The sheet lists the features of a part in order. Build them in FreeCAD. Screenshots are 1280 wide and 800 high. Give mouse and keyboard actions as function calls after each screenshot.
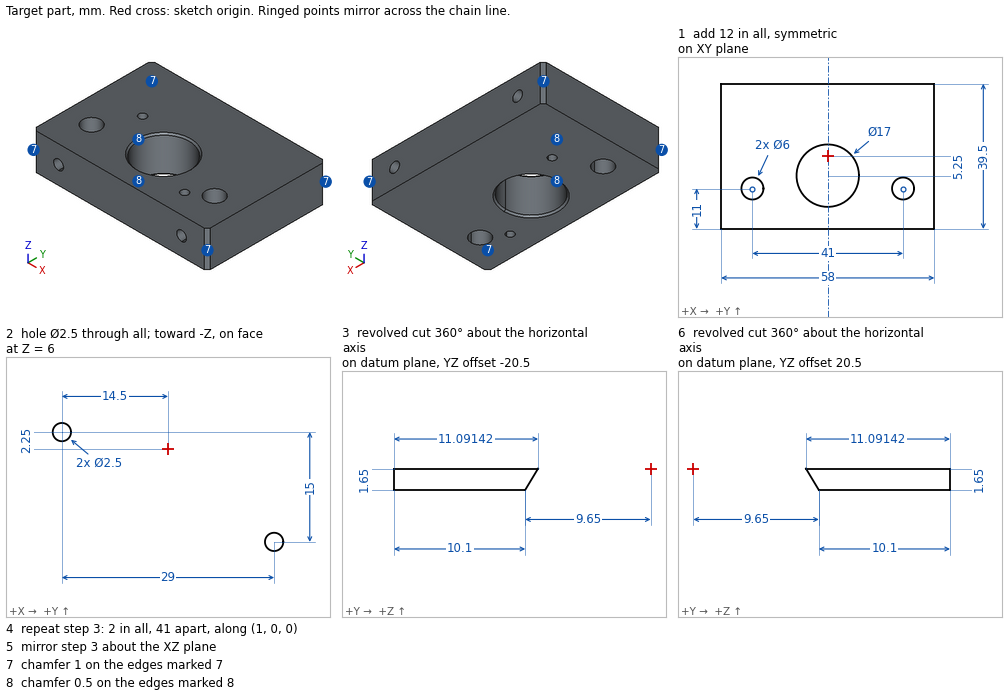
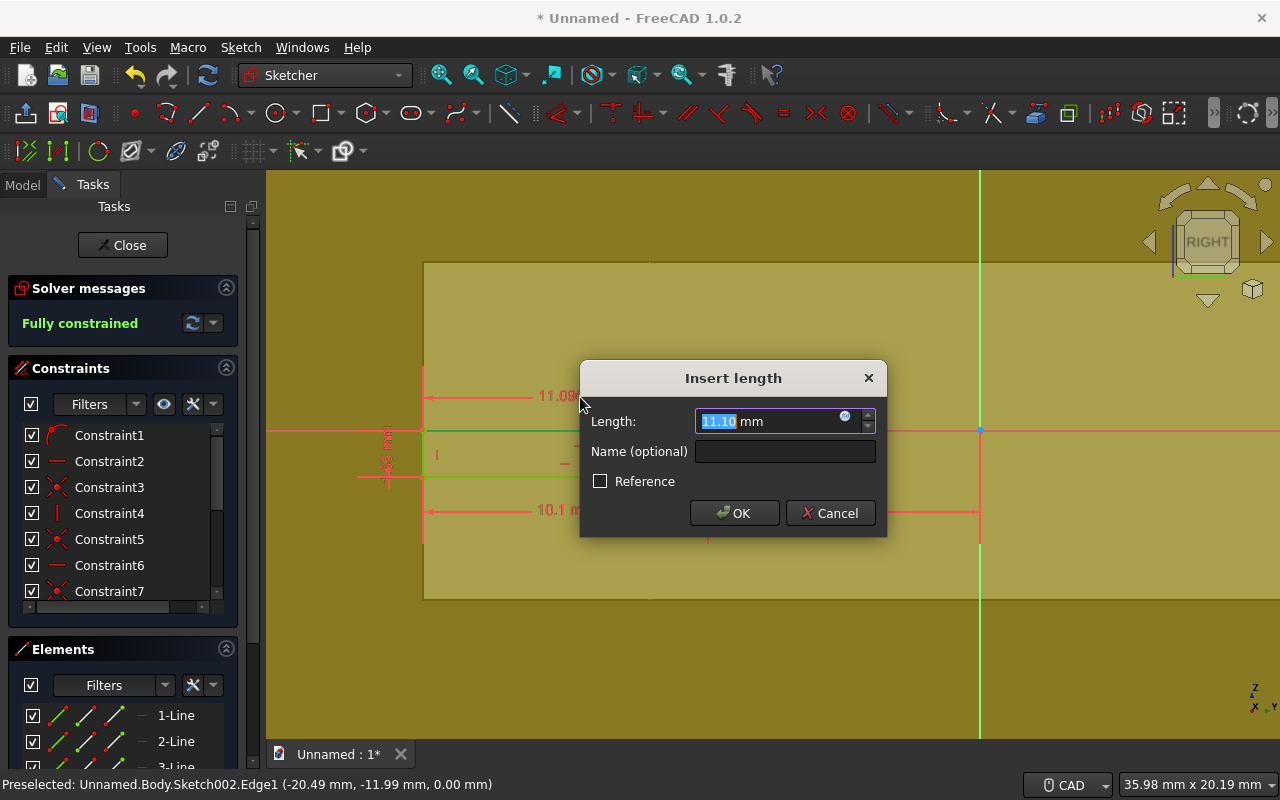
text(11.09142)
key(Return)
key(Escape)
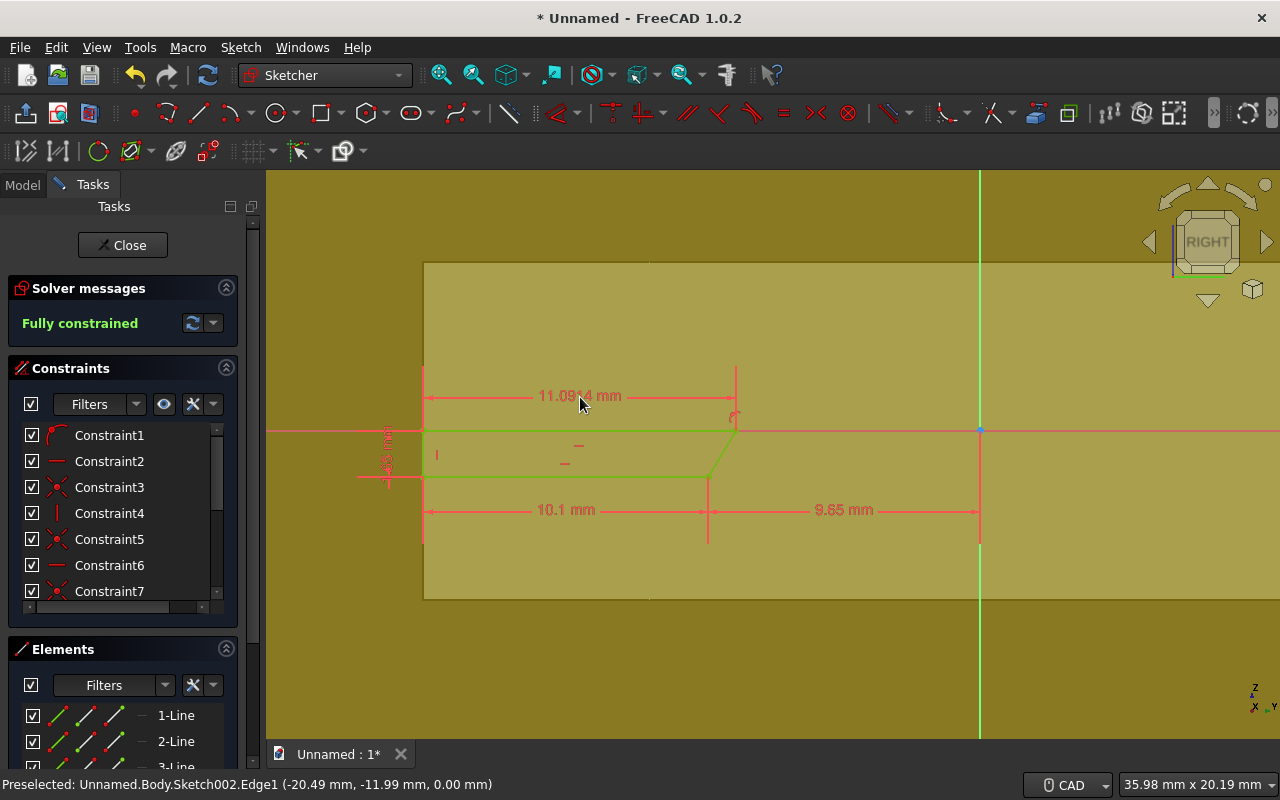
click(123, 245)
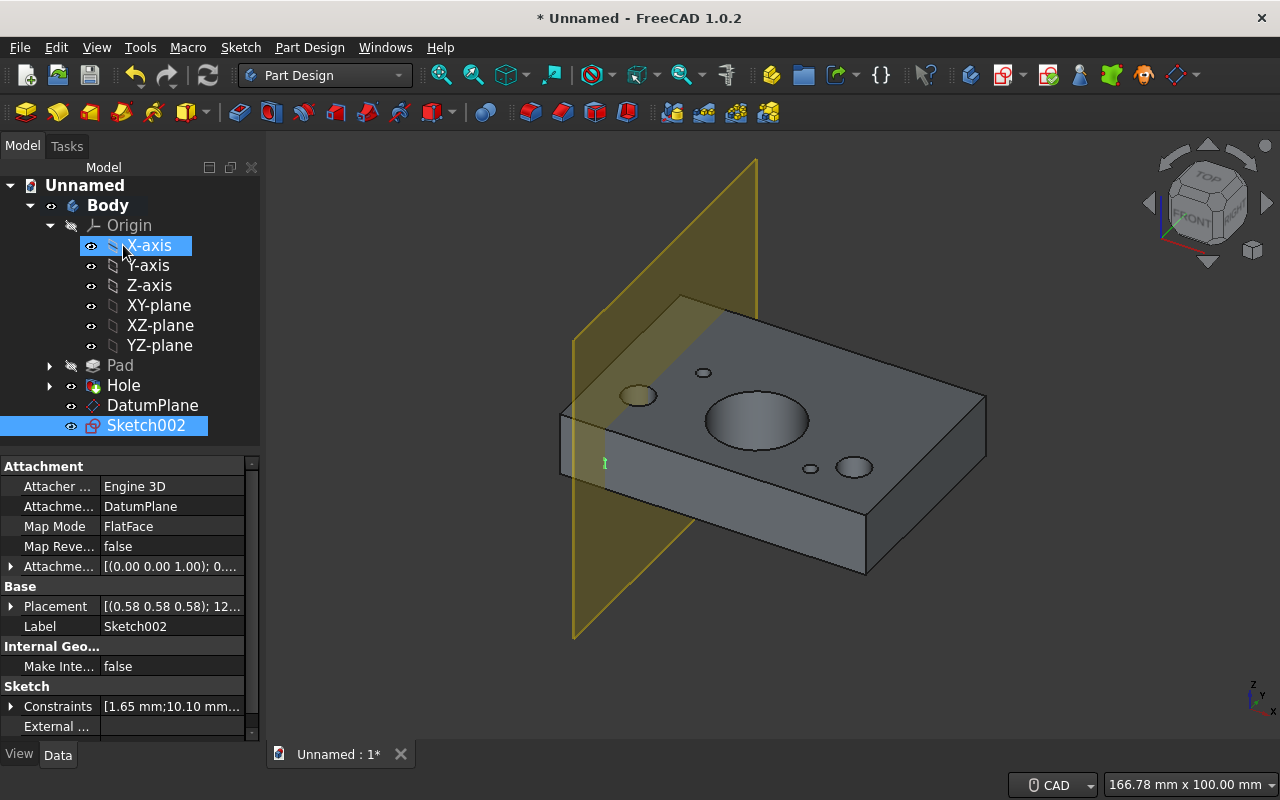
click(304, 112)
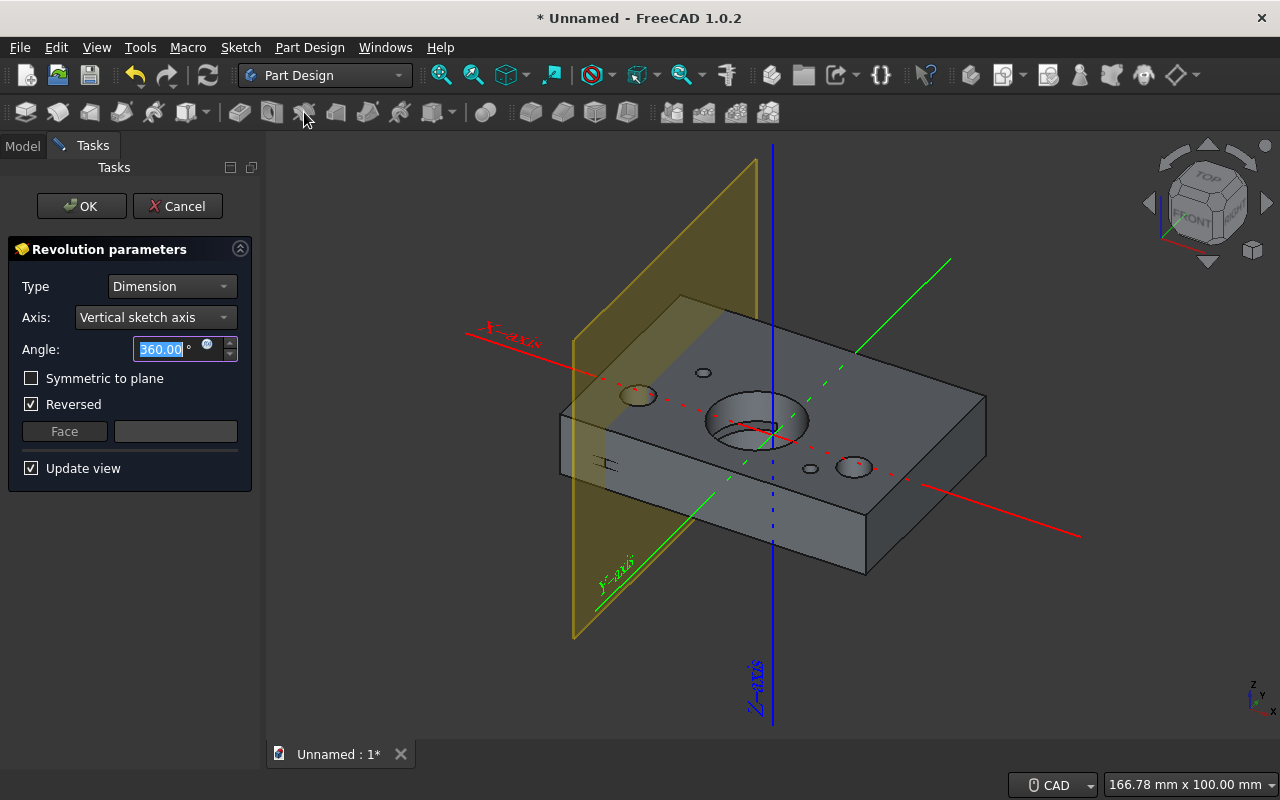
click(156, 318)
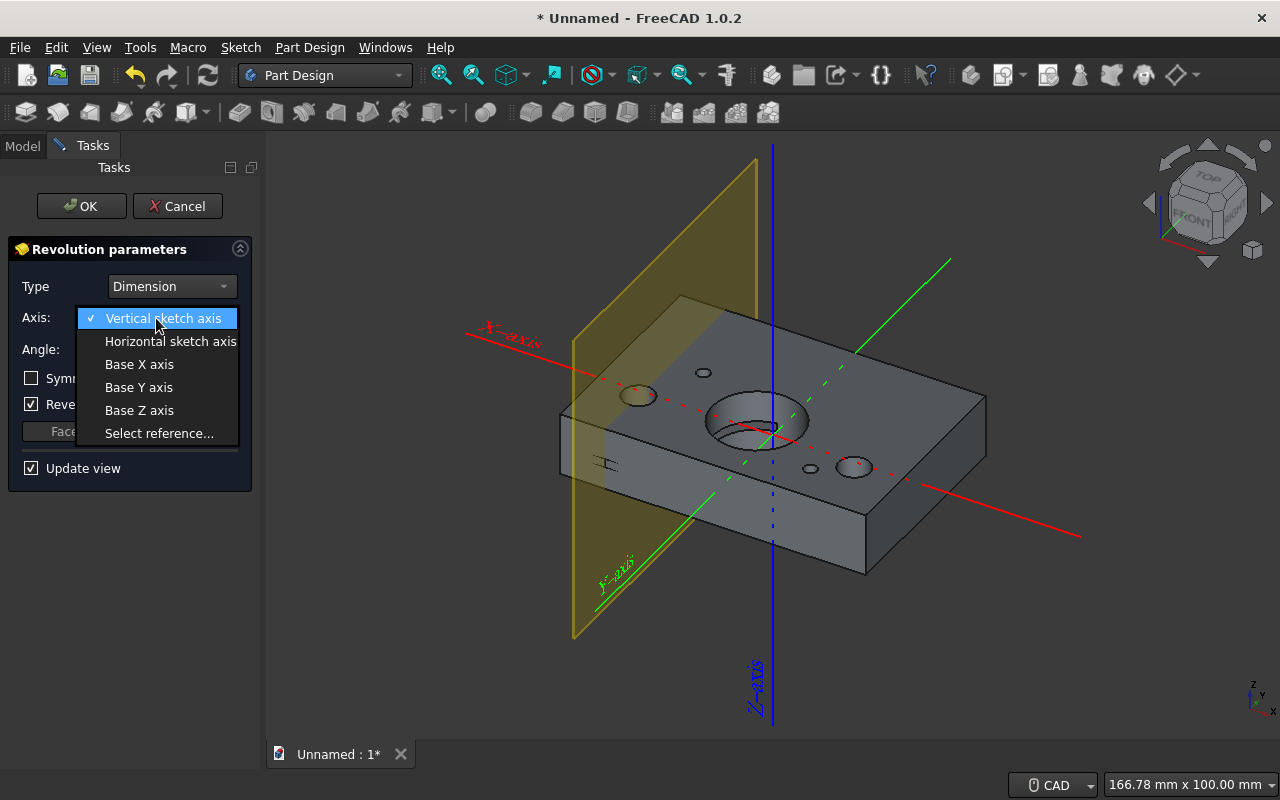
click(156, 342)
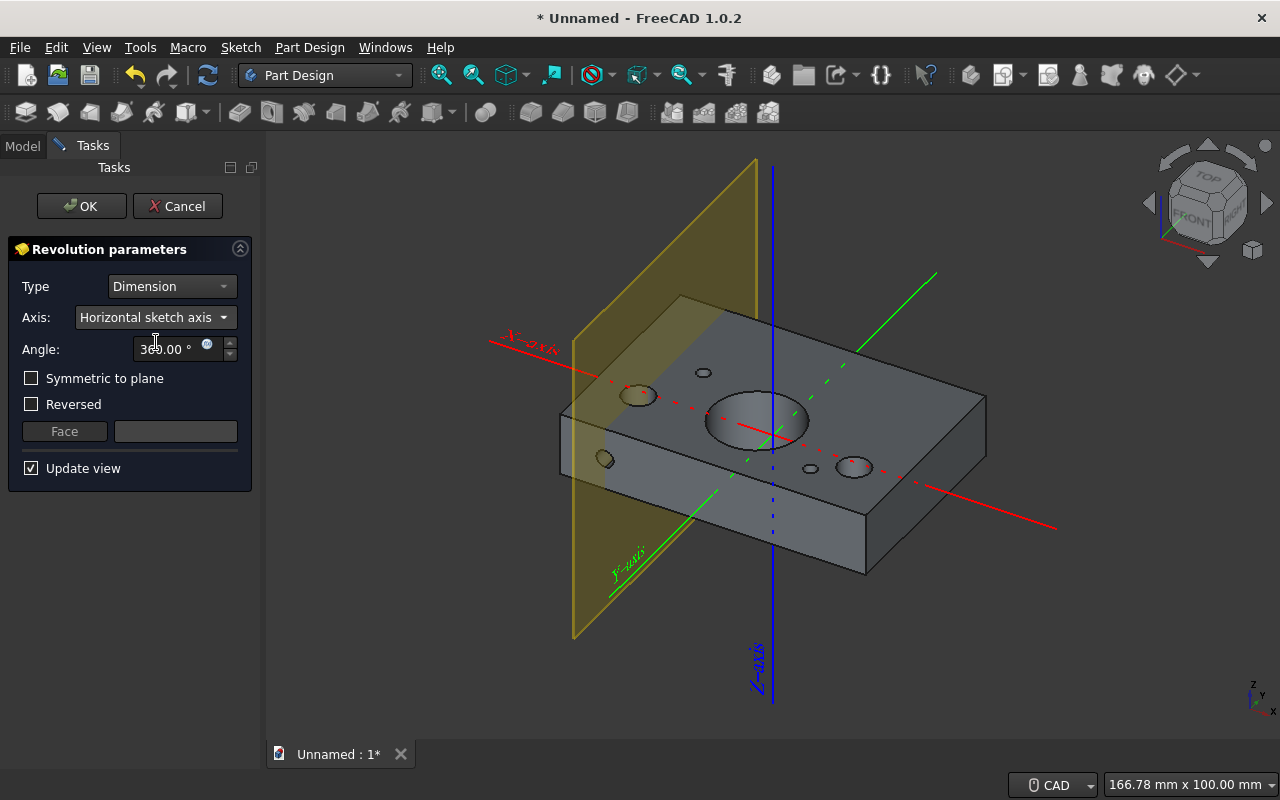
click(82, 206)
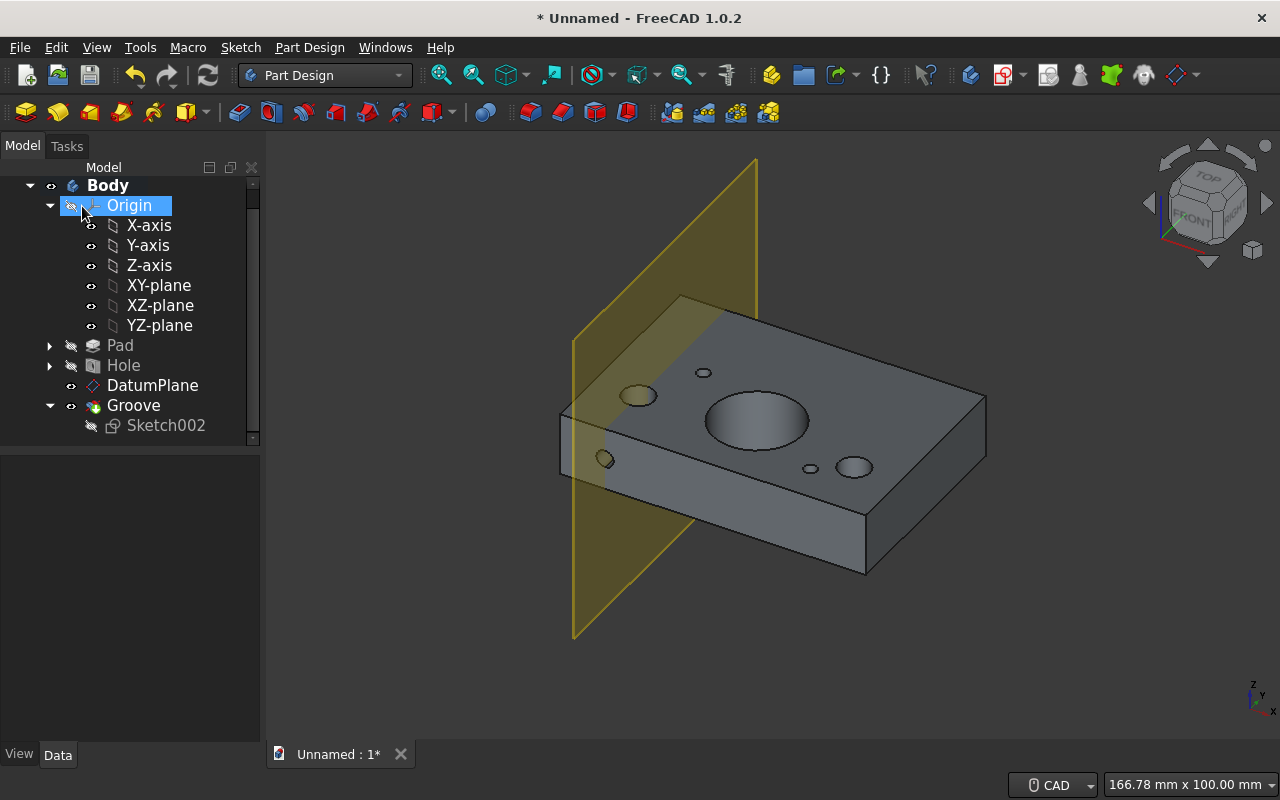
click(116, 386)
key(space)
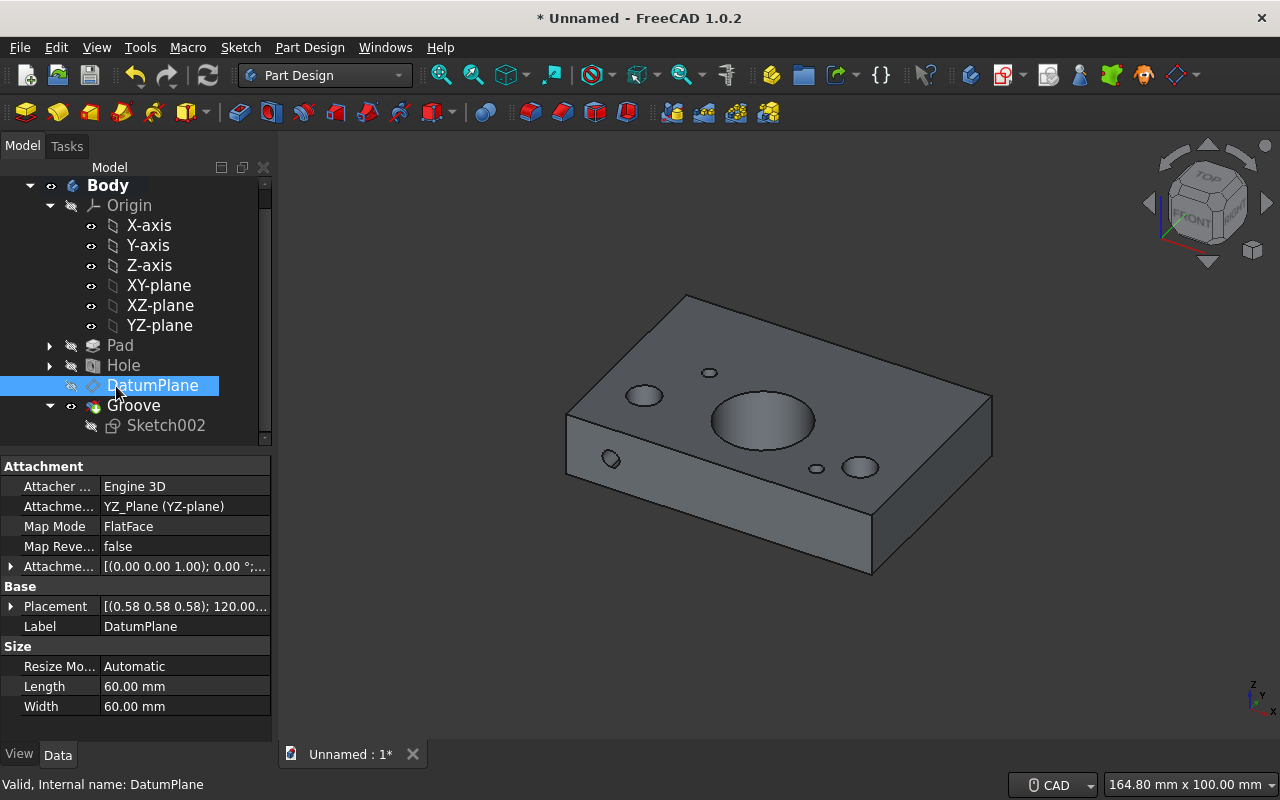
click(116, 406)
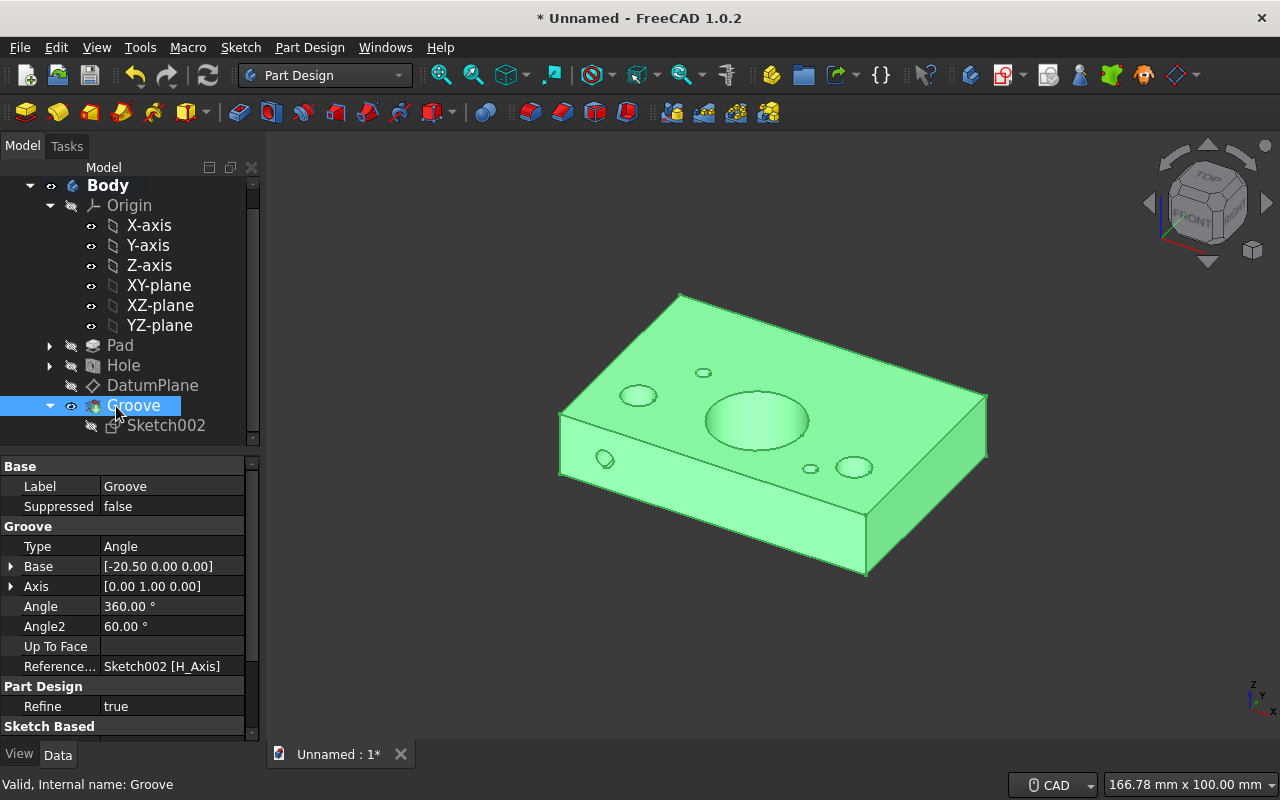
click(704, 112)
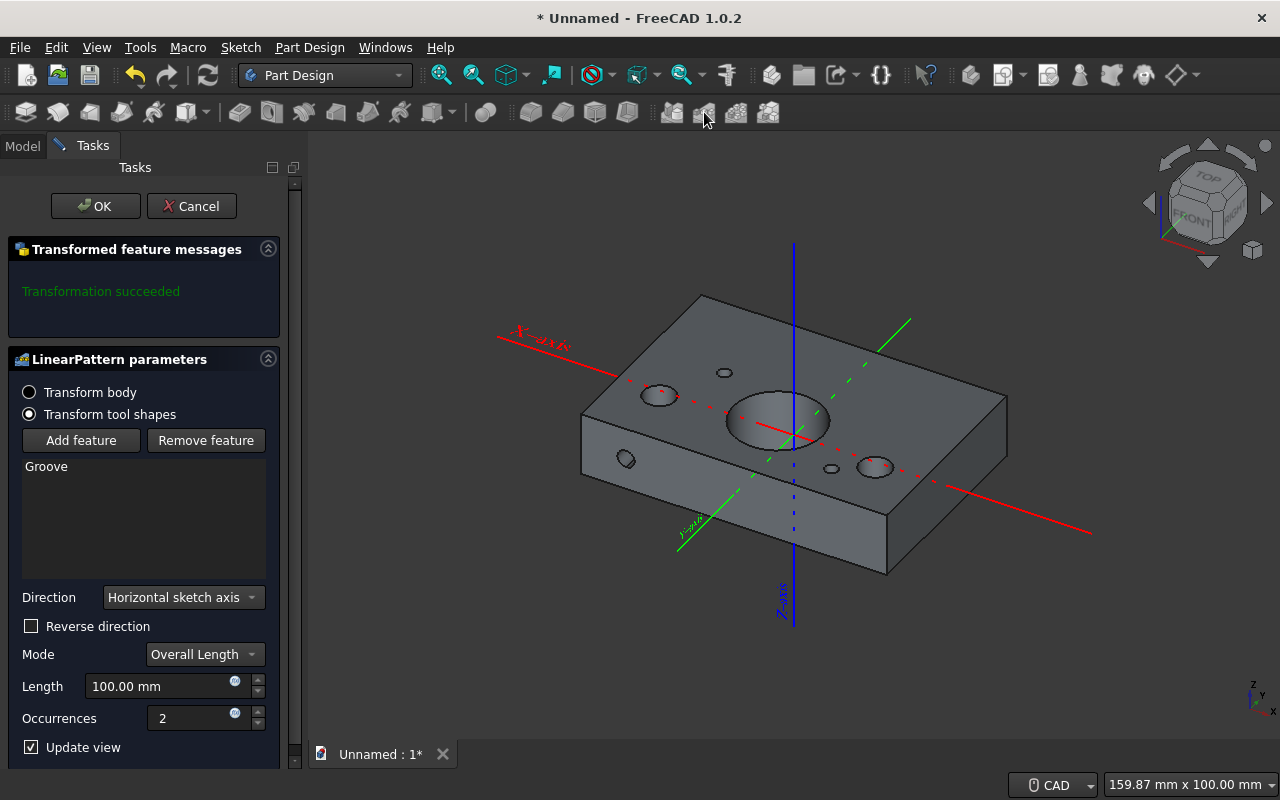
click(184, 598)